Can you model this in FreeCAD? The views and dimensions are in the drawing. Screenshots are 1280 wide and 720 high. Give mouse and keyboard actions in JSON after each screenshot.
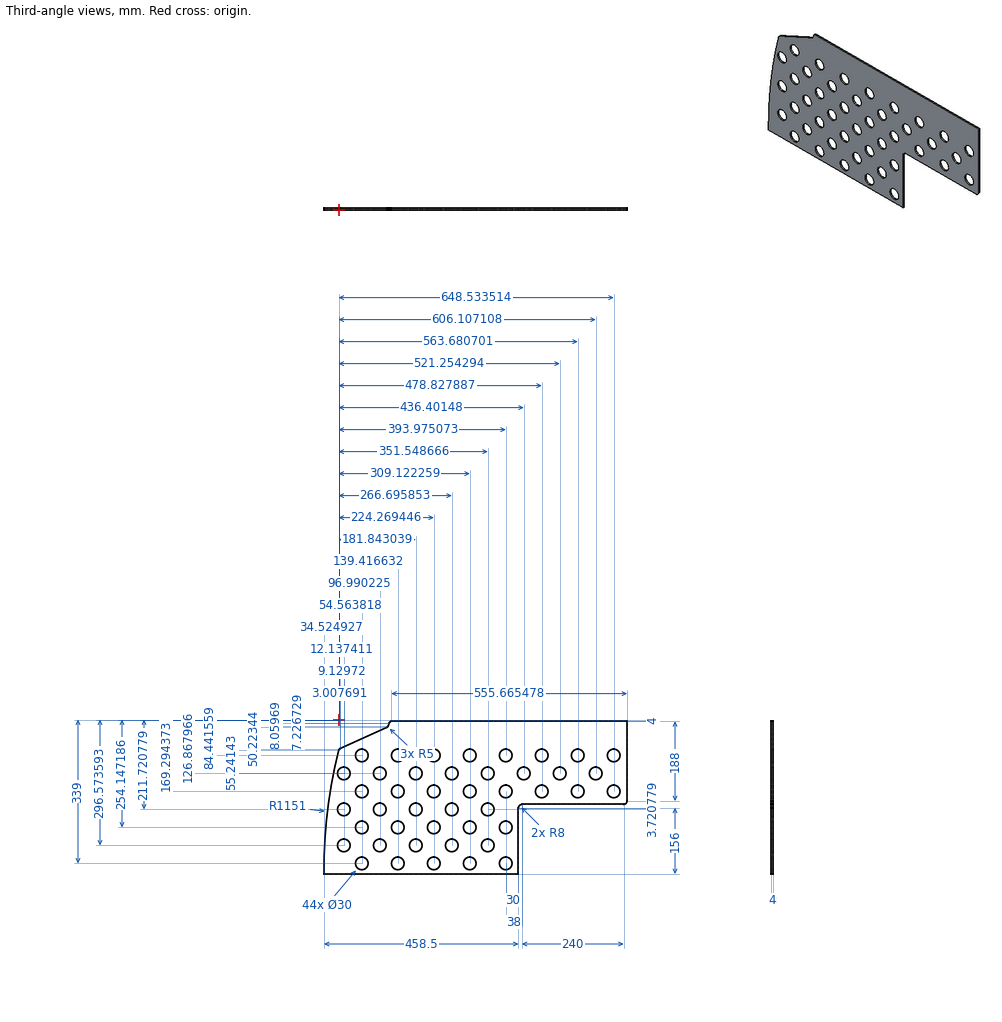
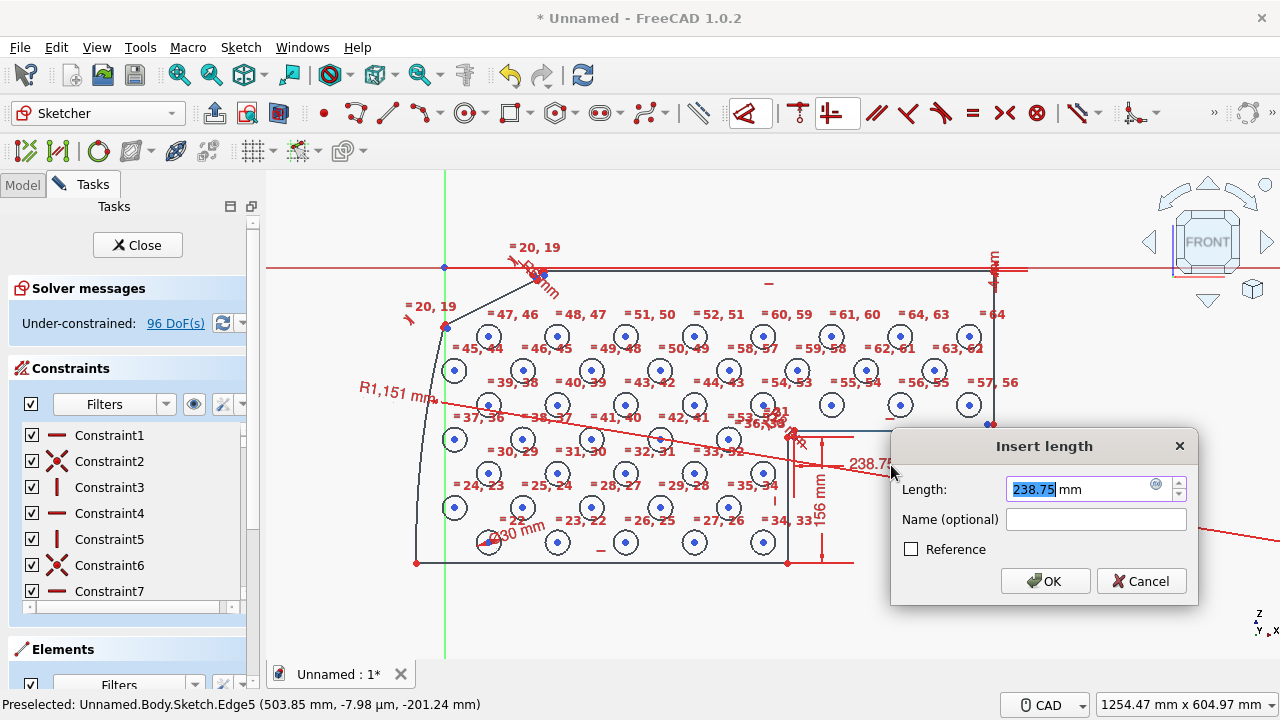
{"action": "type", "text": "240"}
{"action": "key", "text": "Return"}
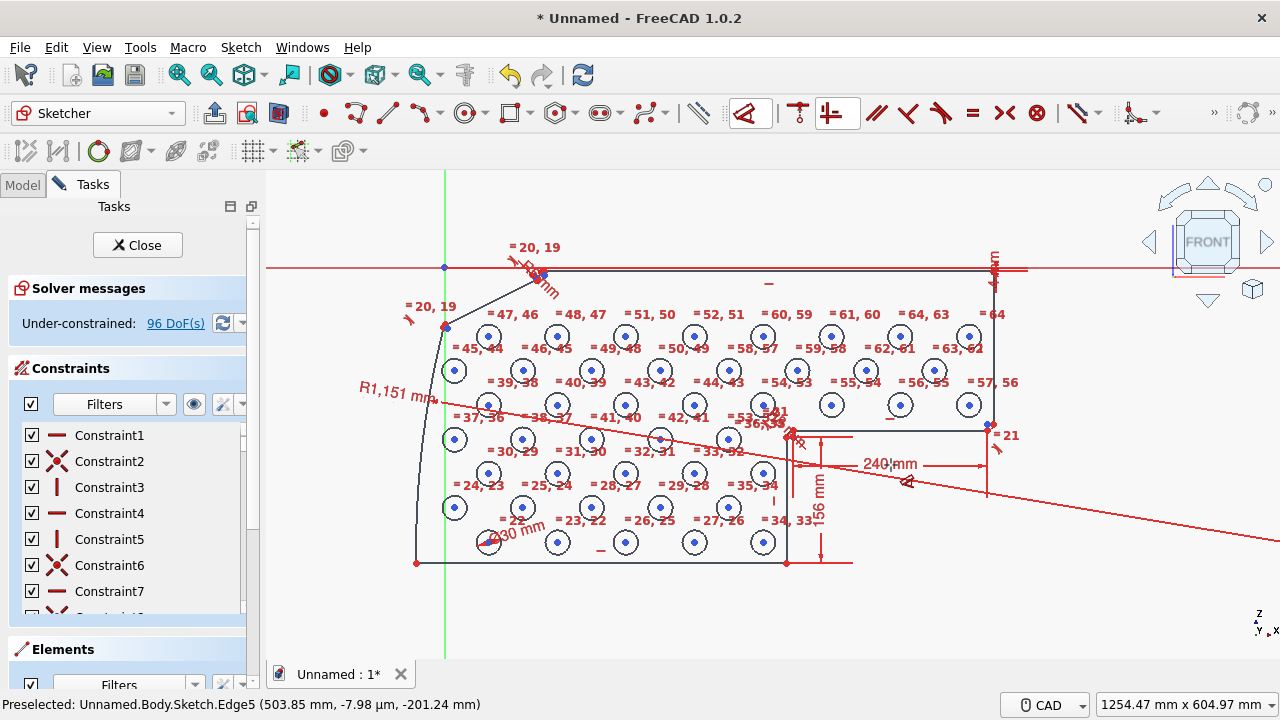
{"action": "left_click", "coordinate": [994, 378]}
{"action": "left_click", "coordinate": [1028, 348]}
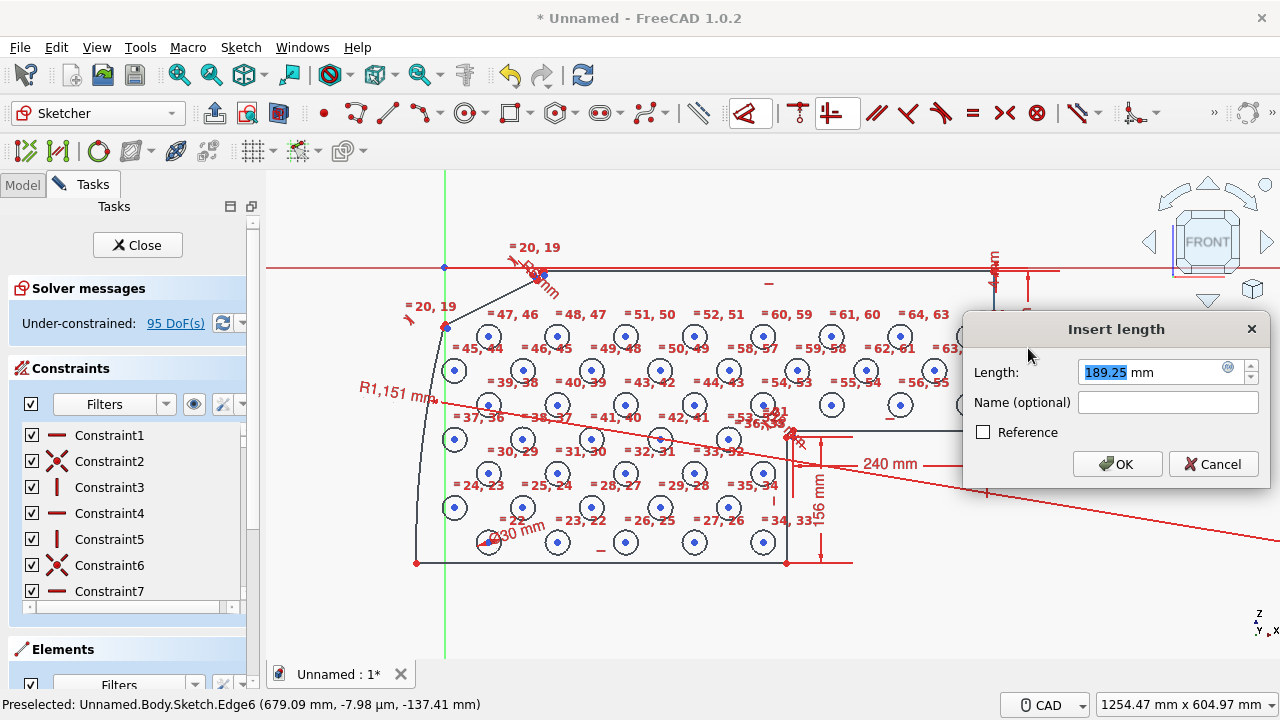
{"action": "type", "text": "188"}
{"action": "key", "text": "Return"}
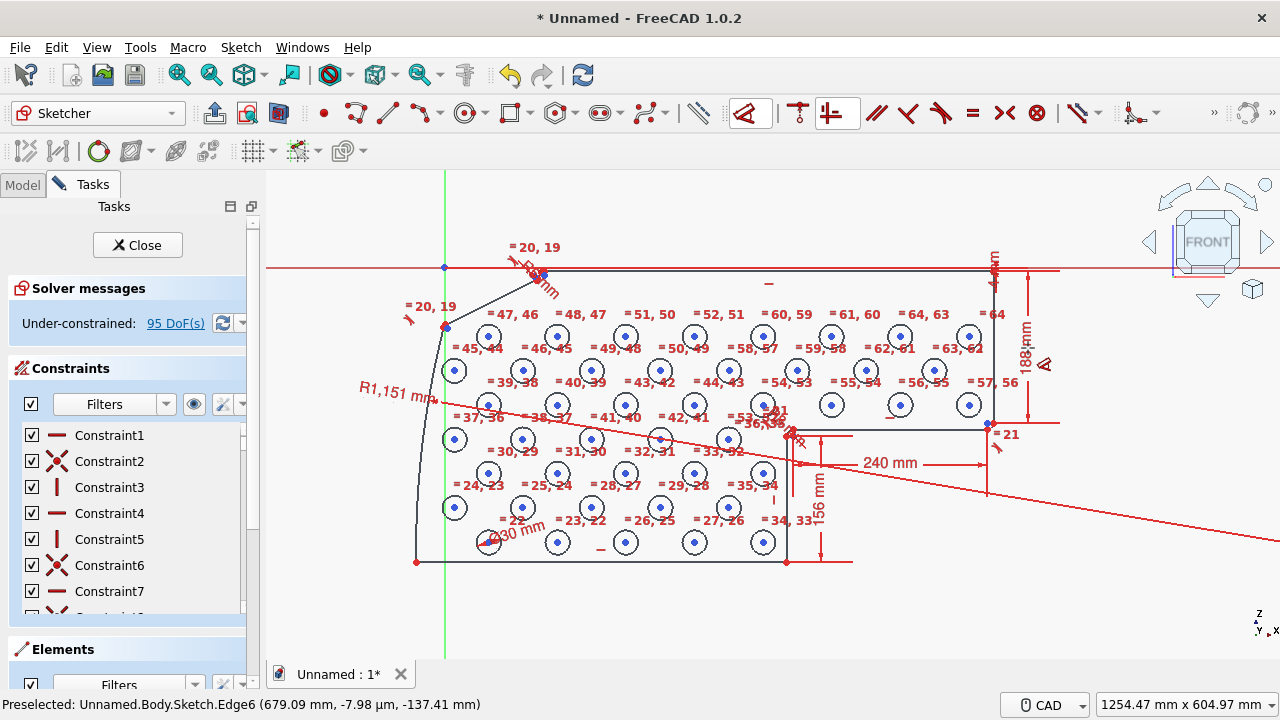
{"action": "left_click", "coordinate": [489, 543]}
{"action": "left_click", "coordinate": [411, 342]}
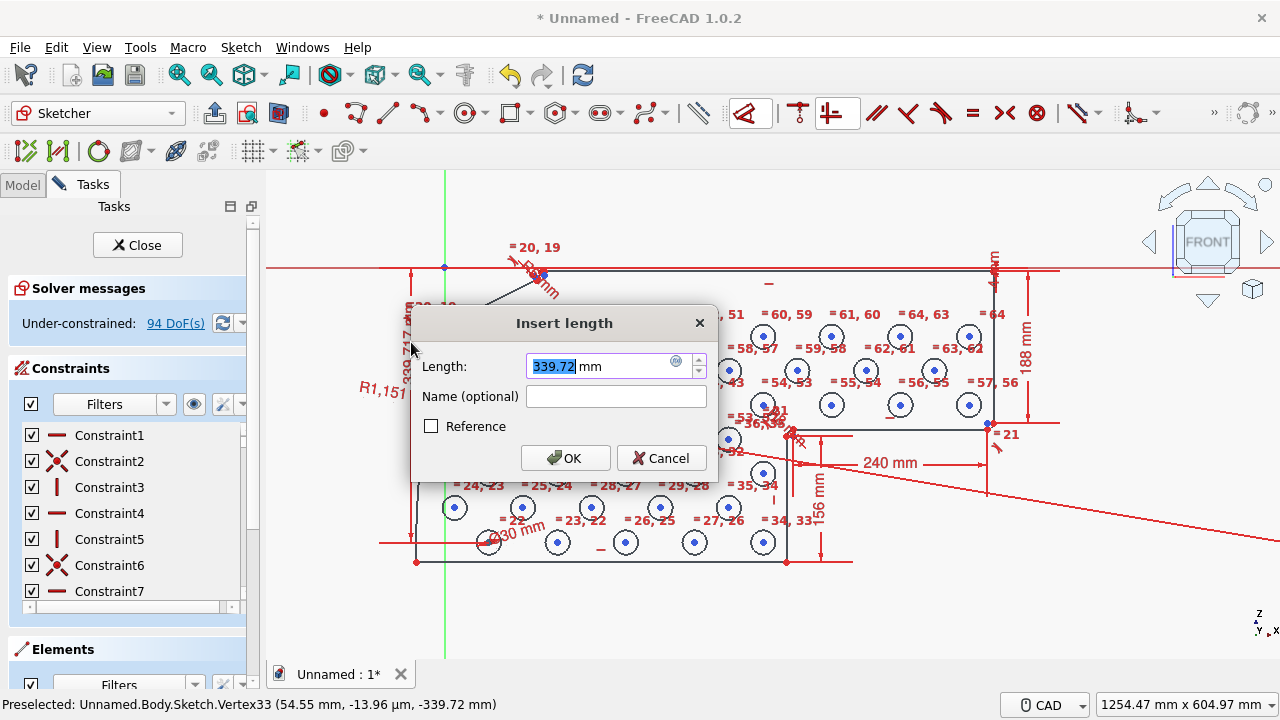
{"action": "type", "text": "339"}
{"action": "key", "text": "Return"}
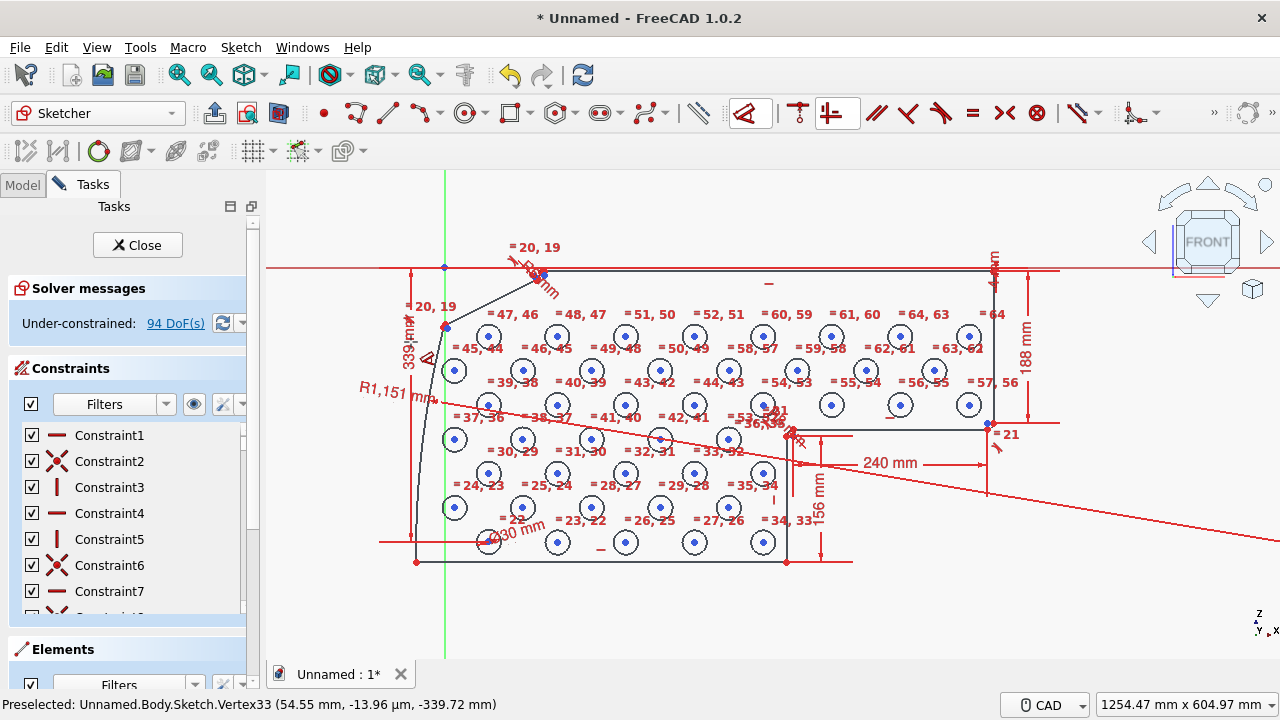
{"action": "left_click", "coordinate": [558, 543]}
{"action": "left_click", "coordinate": [411, 309]}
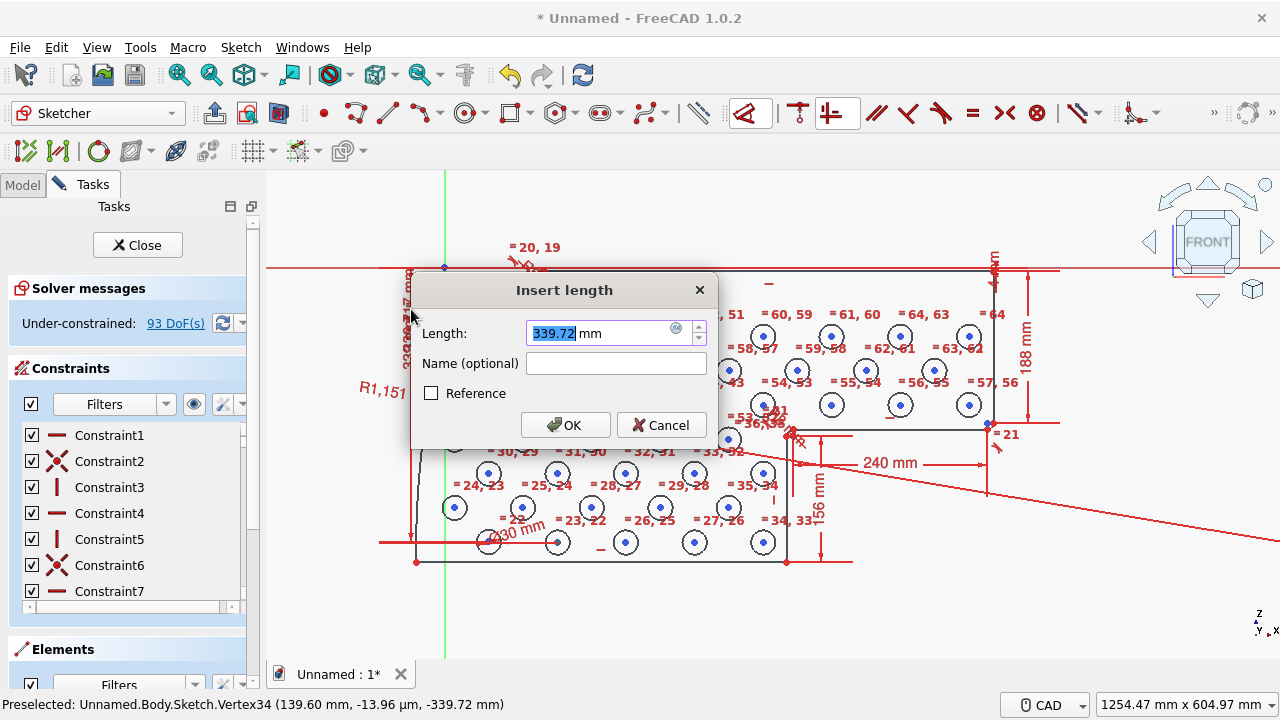
{"action": "type", "text": "339"}
{"action": "key", "text": "Return"}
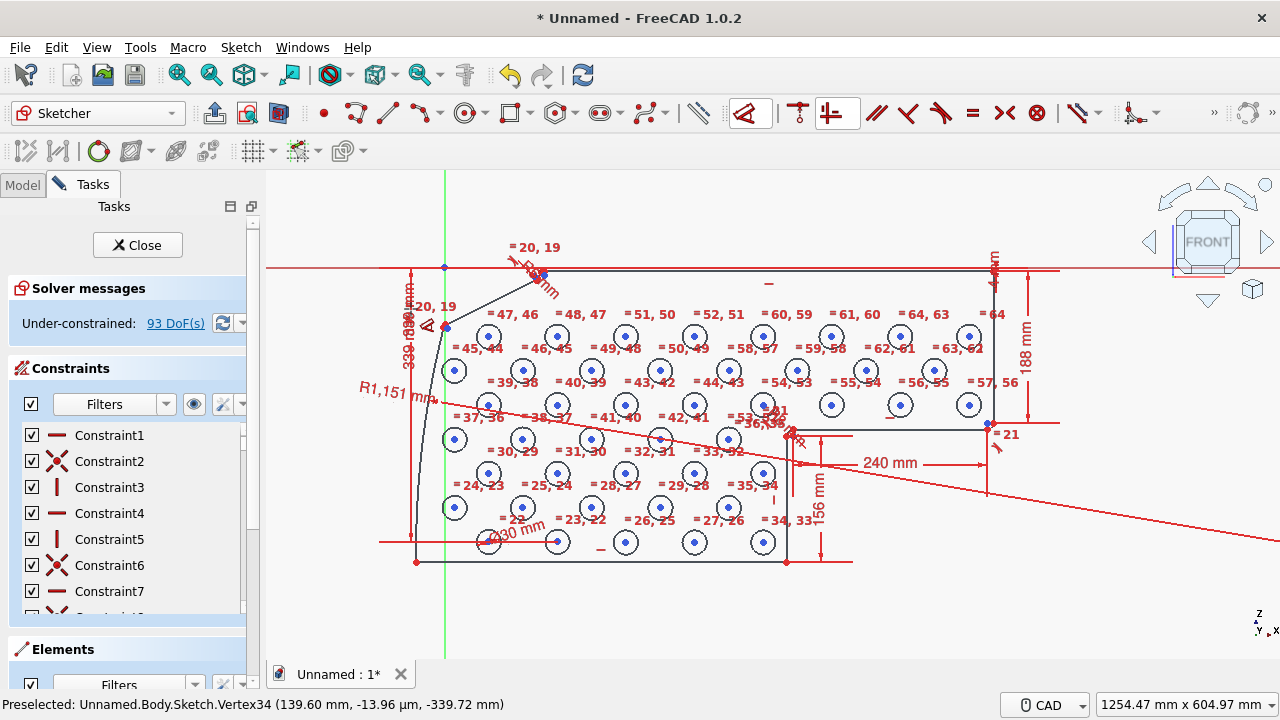
{"action": "left_click", "coordinate": [626, 543]}
{"action": "left_click", "coordinate": [660, 405]}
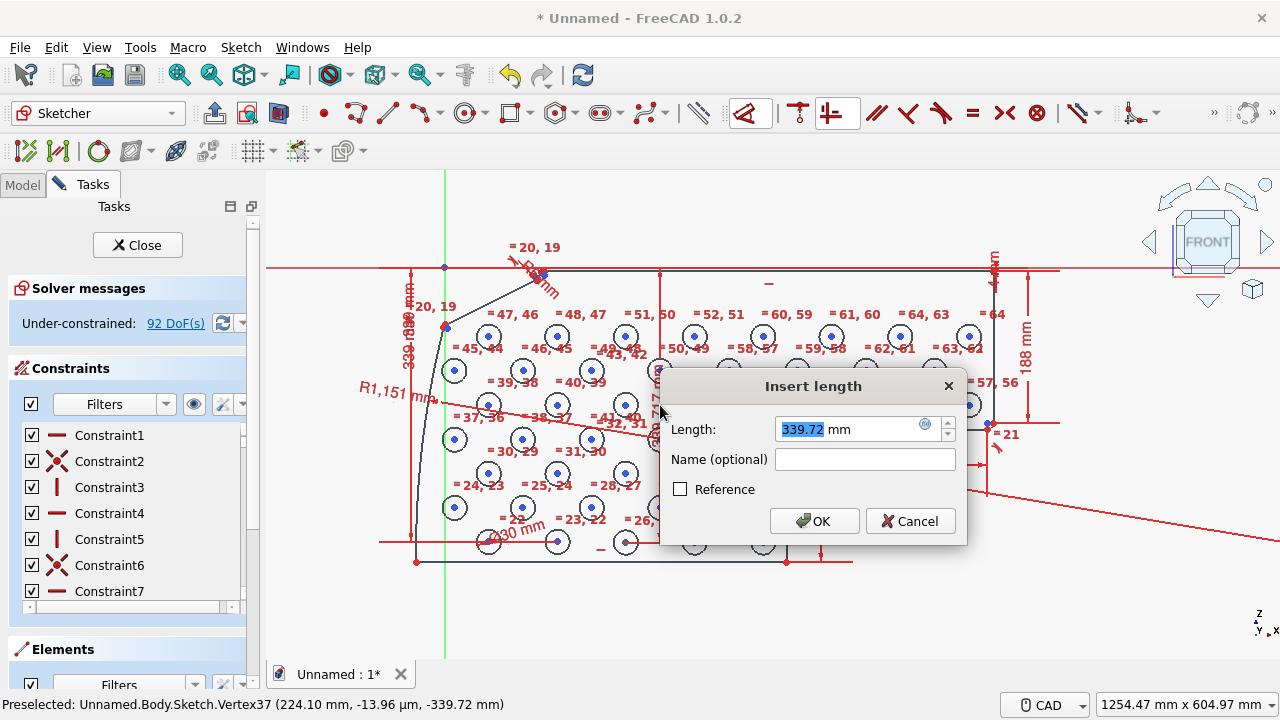
{"action": "type", "text": "339"}
{"action": "key", "text": "Return"}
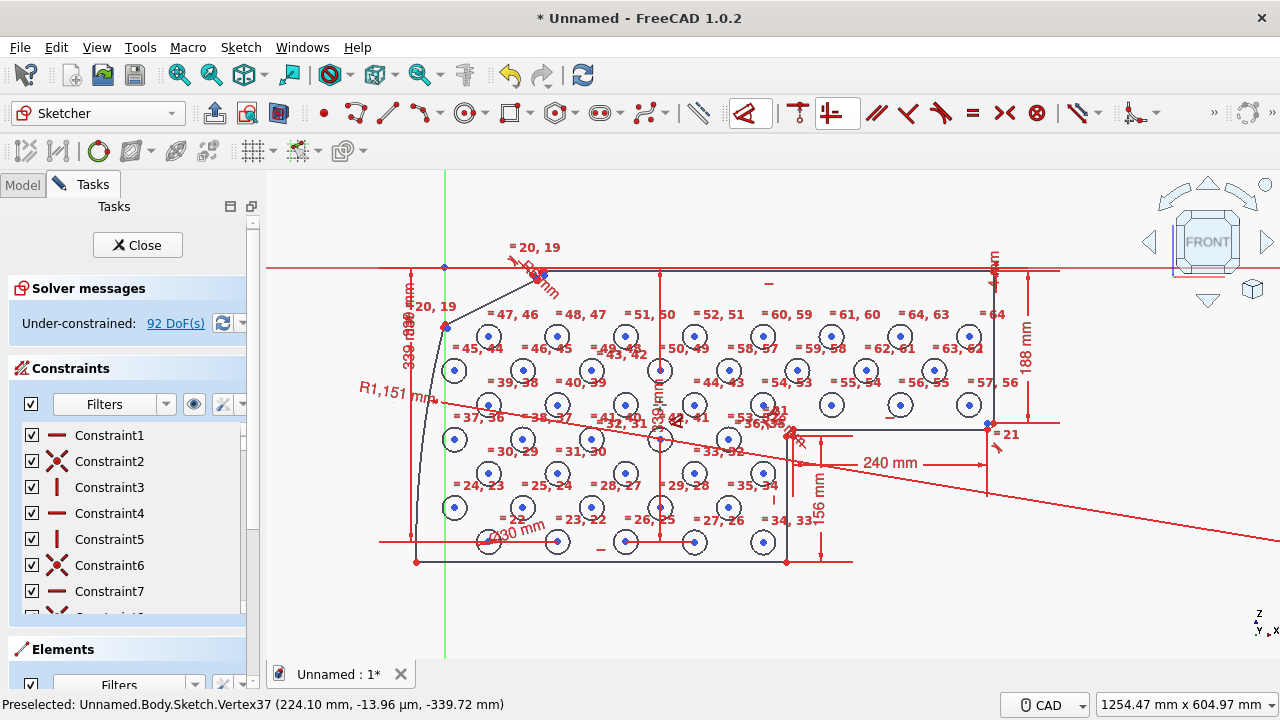
{"action": "left_click", "coordinate": [695, 543]}
{"action": "left_click", "coordinate": [729, 342]}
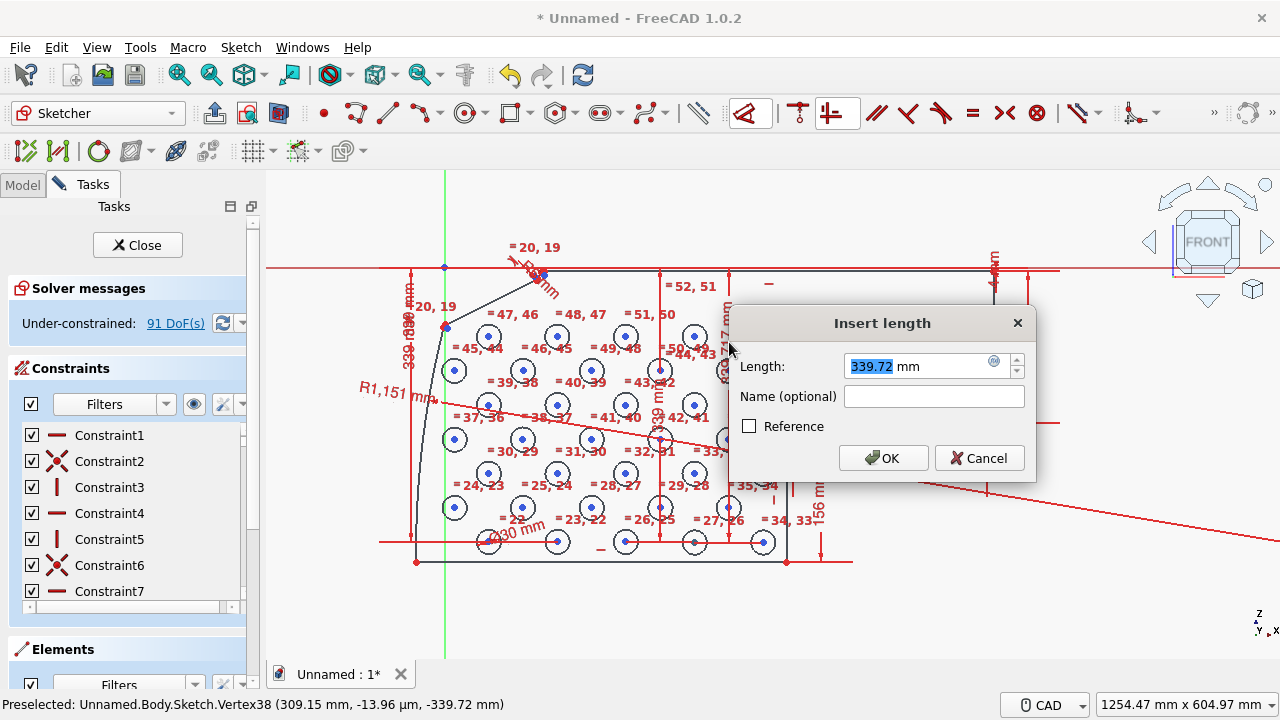
{"action": "type", "text": "339"}
{"action": "key", "text": "Return"}